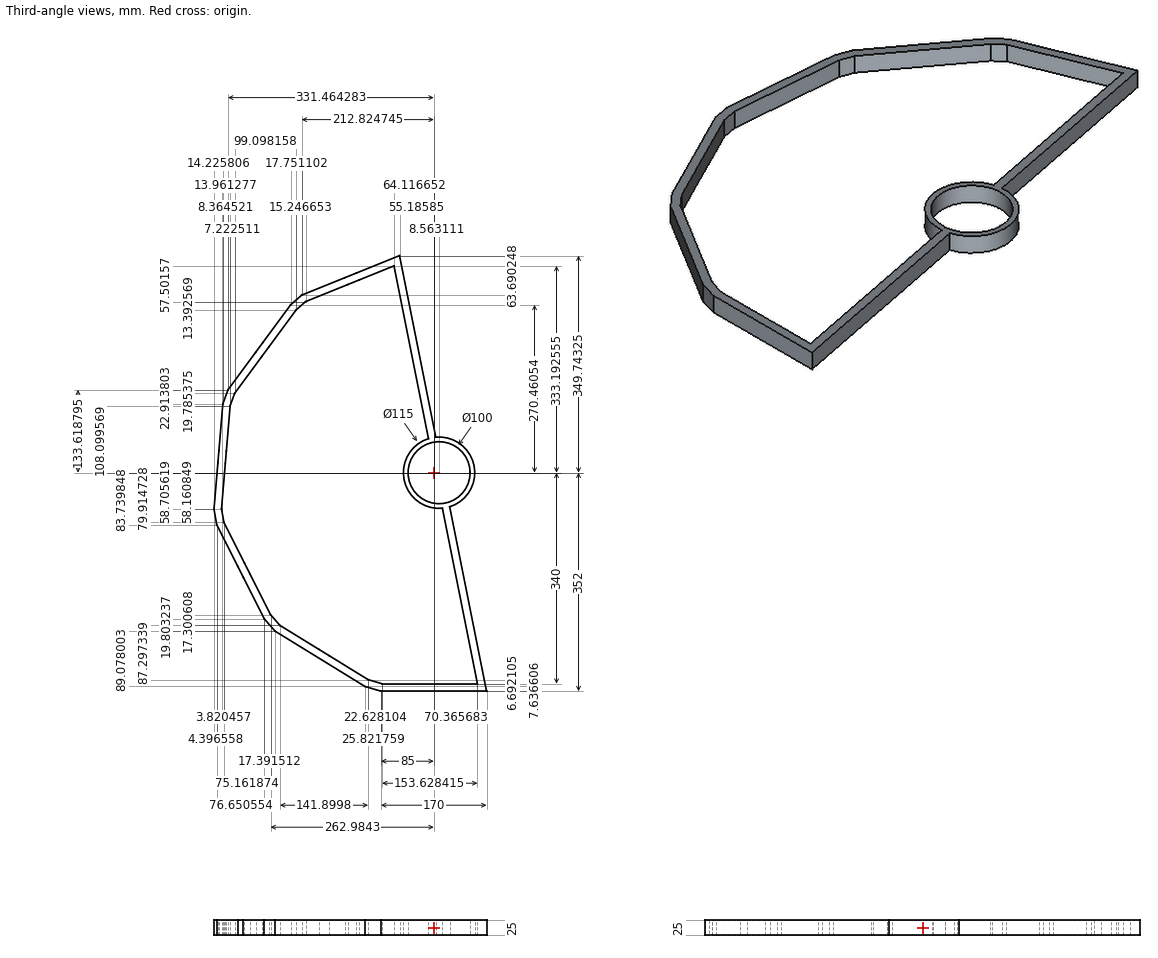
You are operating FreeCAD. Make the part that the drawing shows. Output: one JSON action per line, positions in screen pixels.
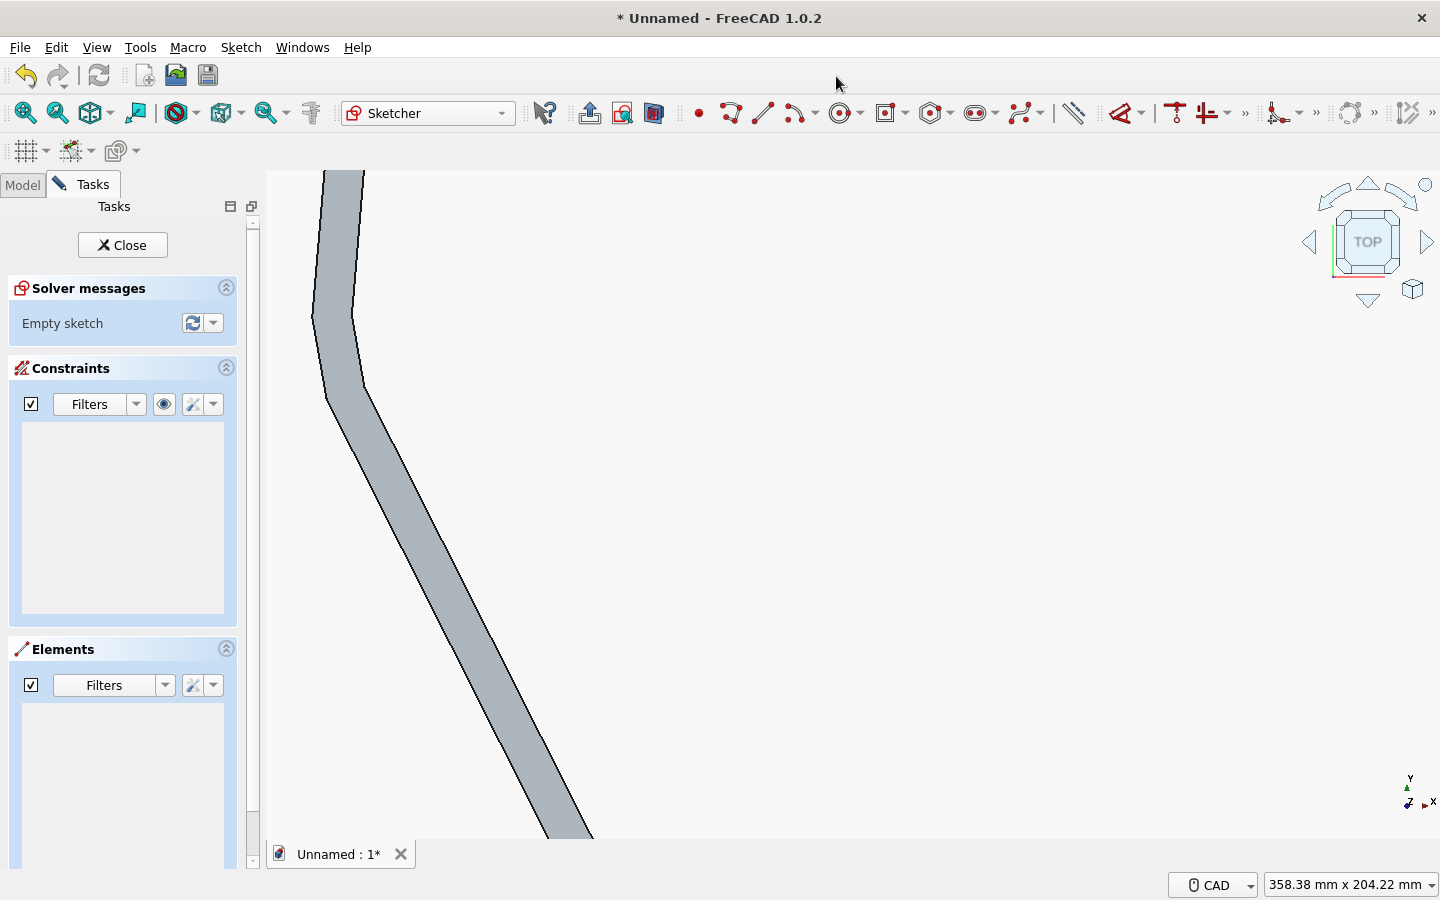
{"action": "scroll", "coordinate": [294, 811], "scroll_direction": "down", "scroll_amount": 2}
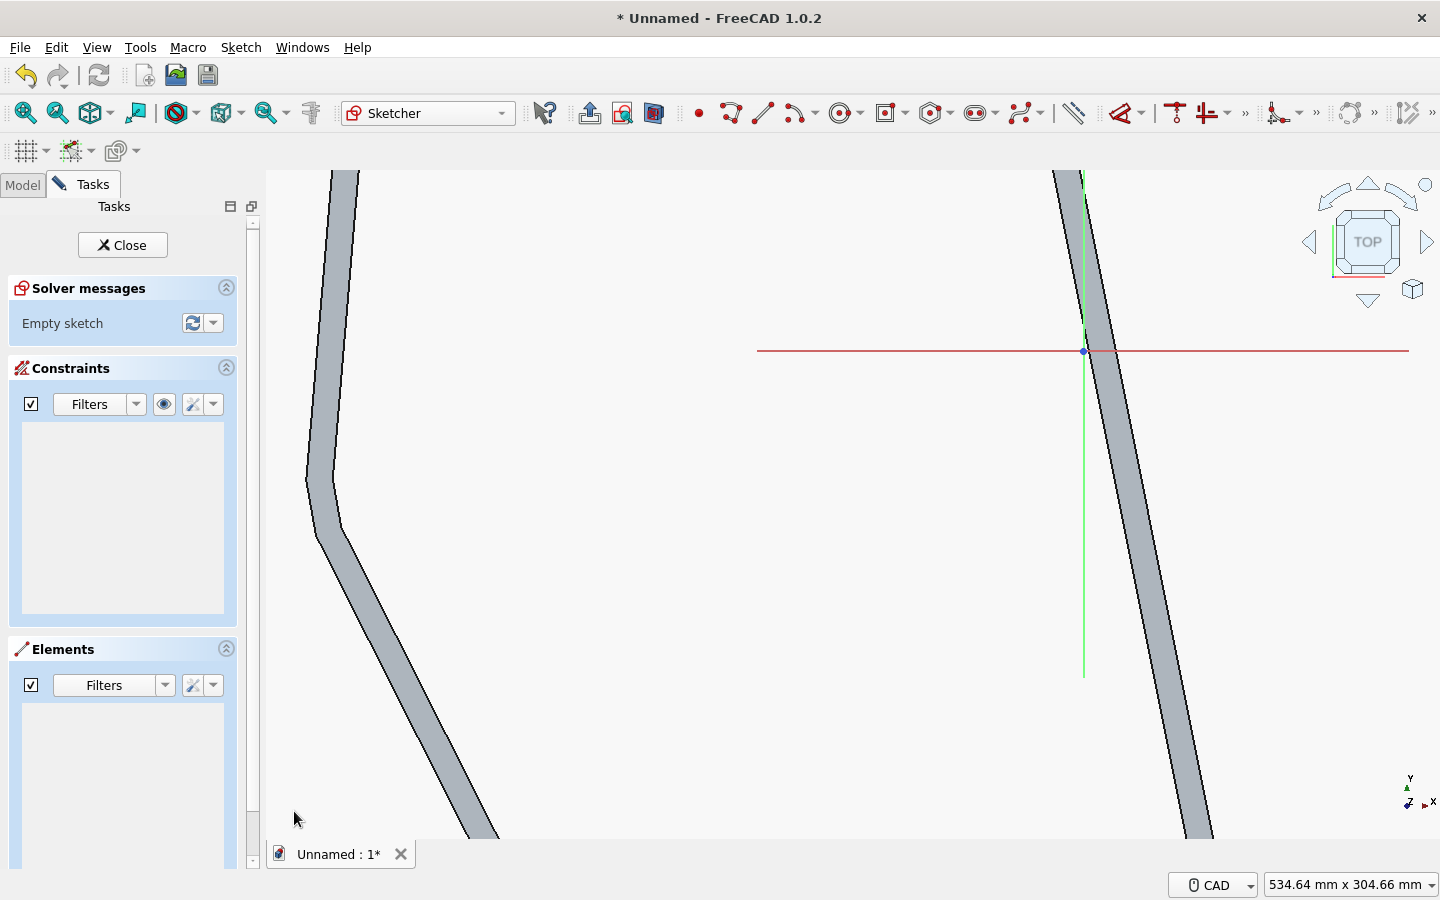
{"action": "scroll", "coordinate": [1275, 198], "scroll_direction": "up", "scroll_amount": 3}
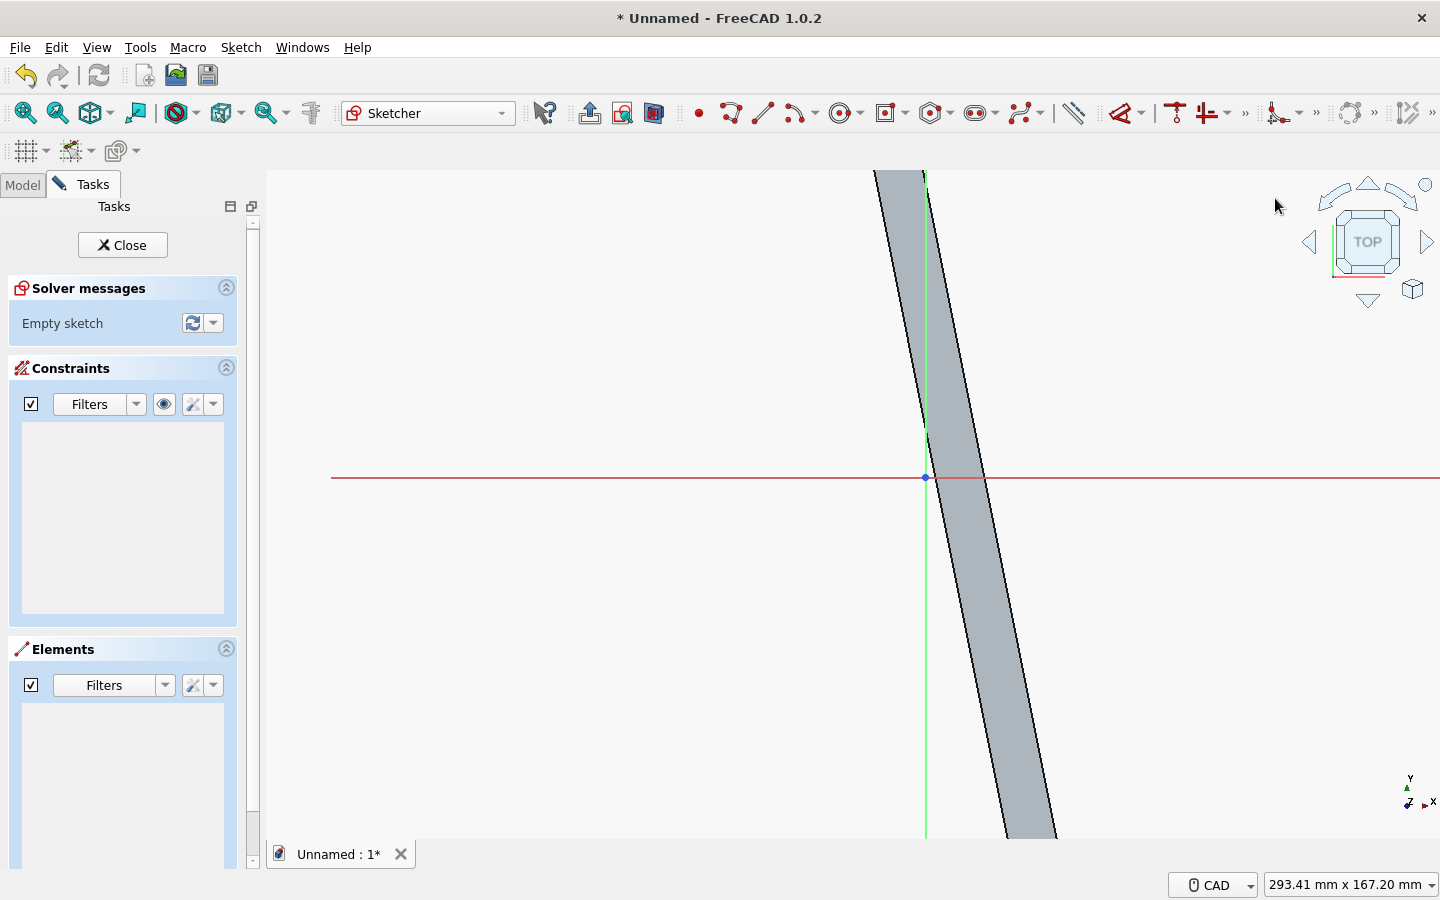
{"action": "left_click", "coordinate": [840, 114]}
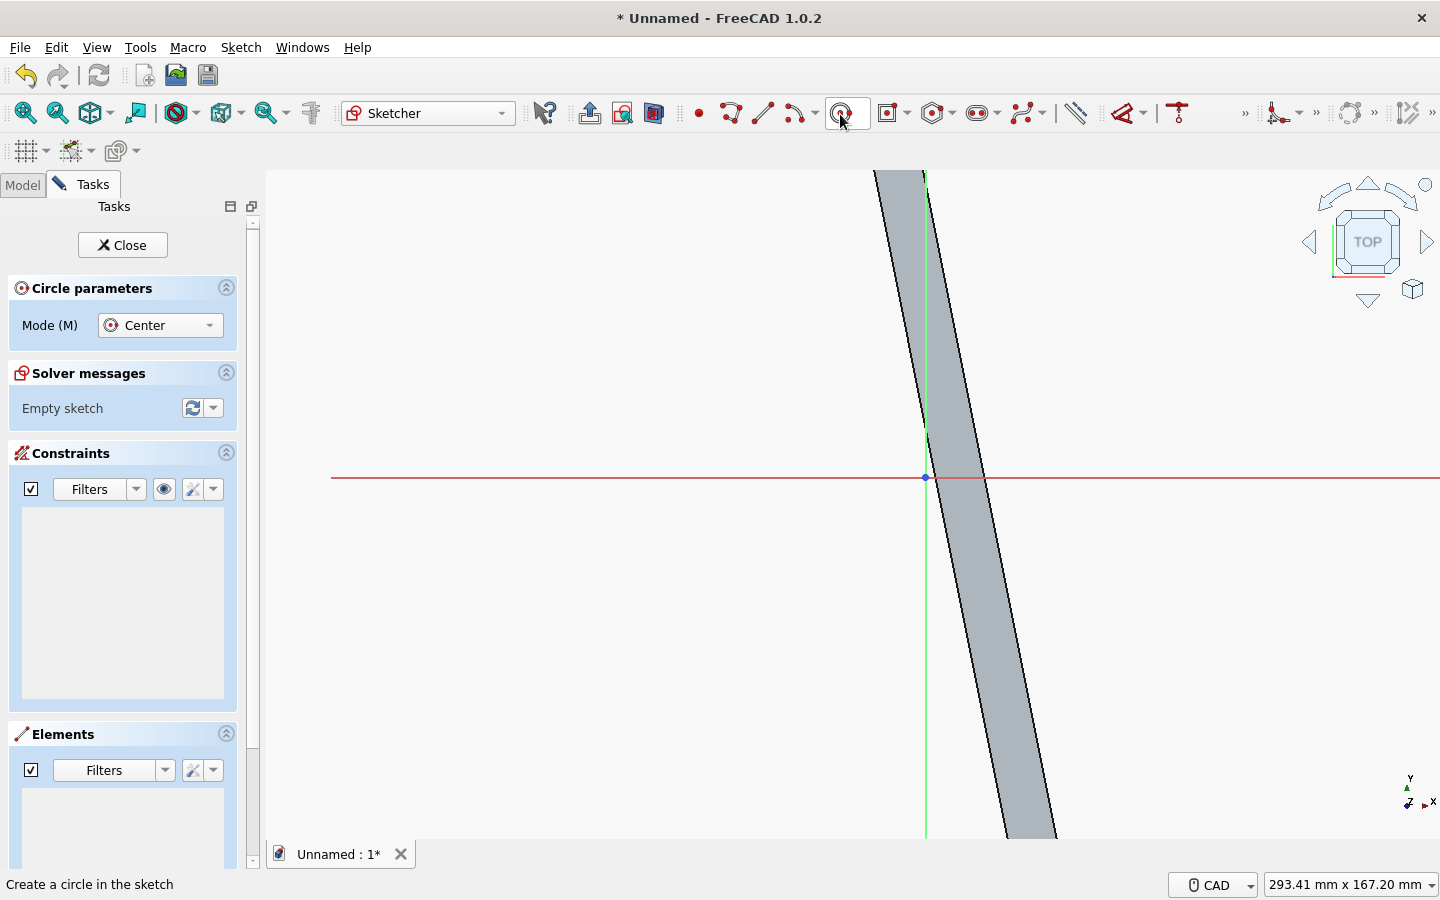
{"action": "left_click", "coordinate": [960, 478]}
{"action": "left_click", "coordinate": [1101, 336]}
{"action": "key", "text": "Escape"}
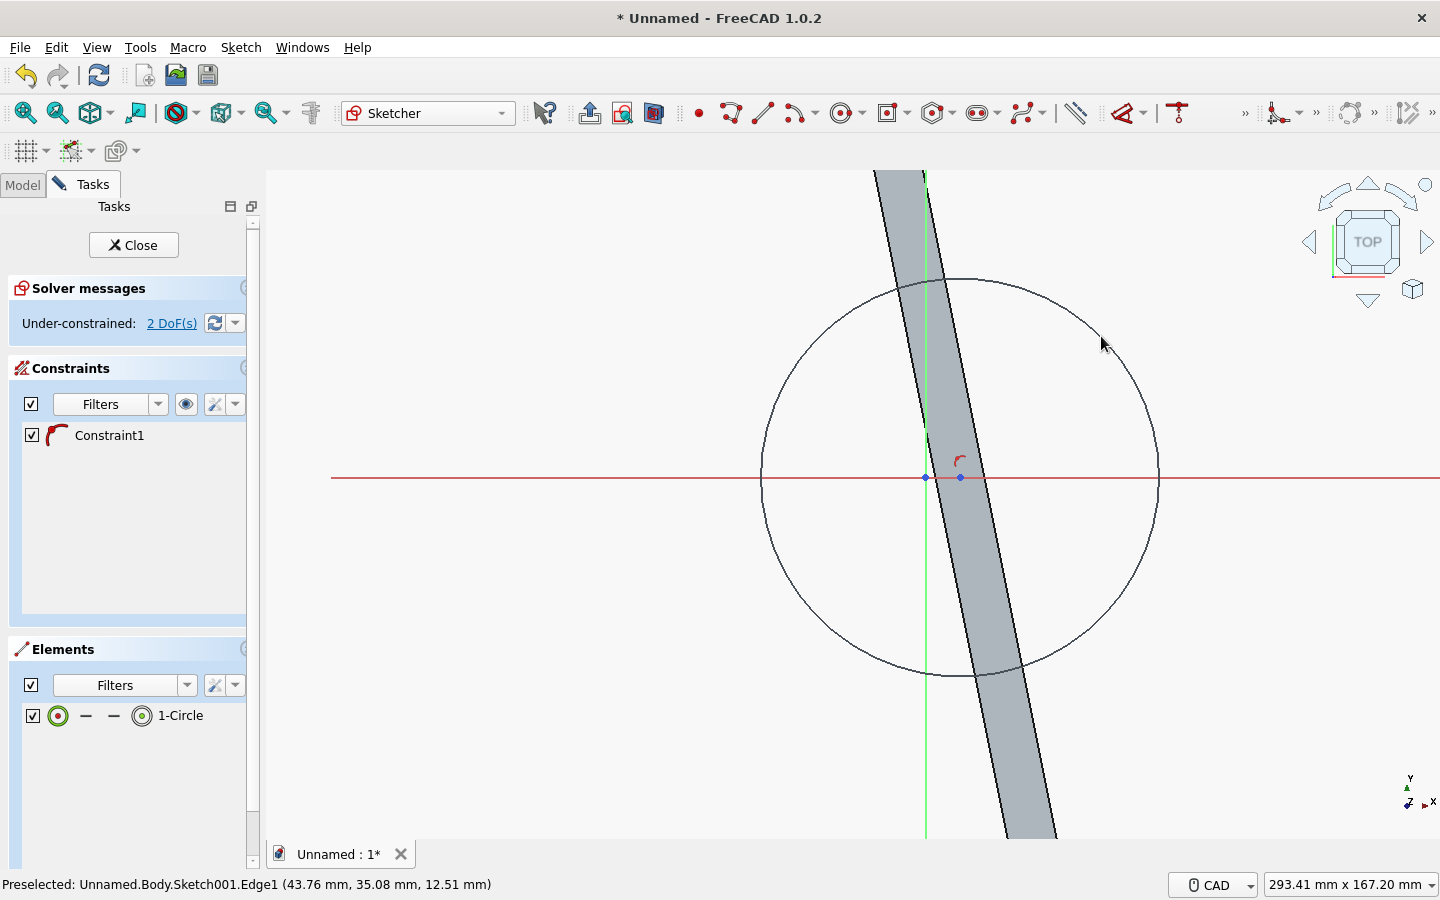
{"action": "left_click", "coordinate": [1122, 114]}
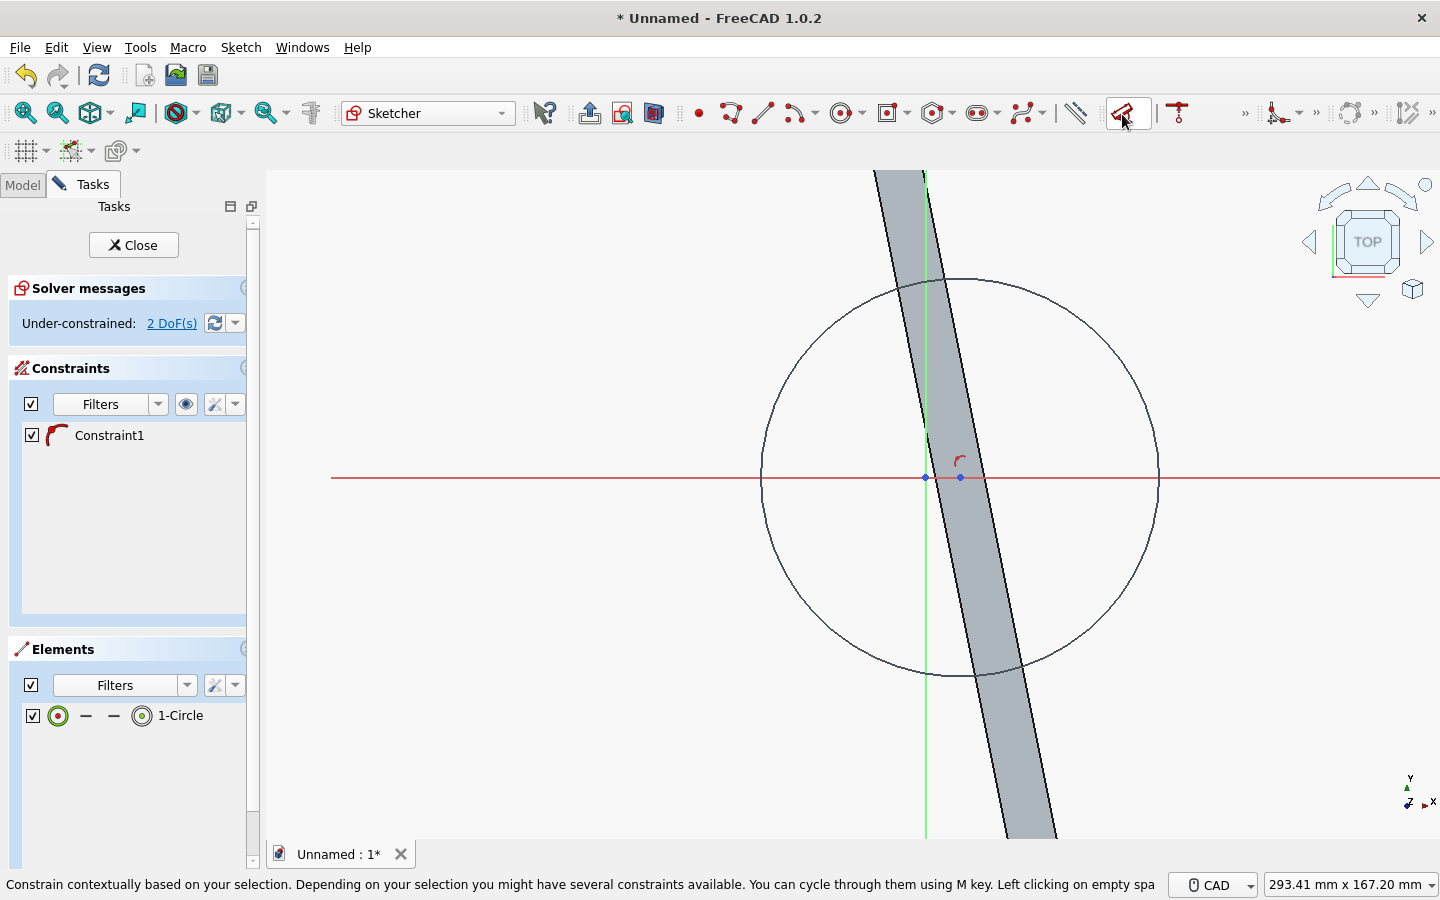
{"action": "left_click", "coordinate": [1100, 336]}
{"action": "left_click", "coordinate": [1122, 313]}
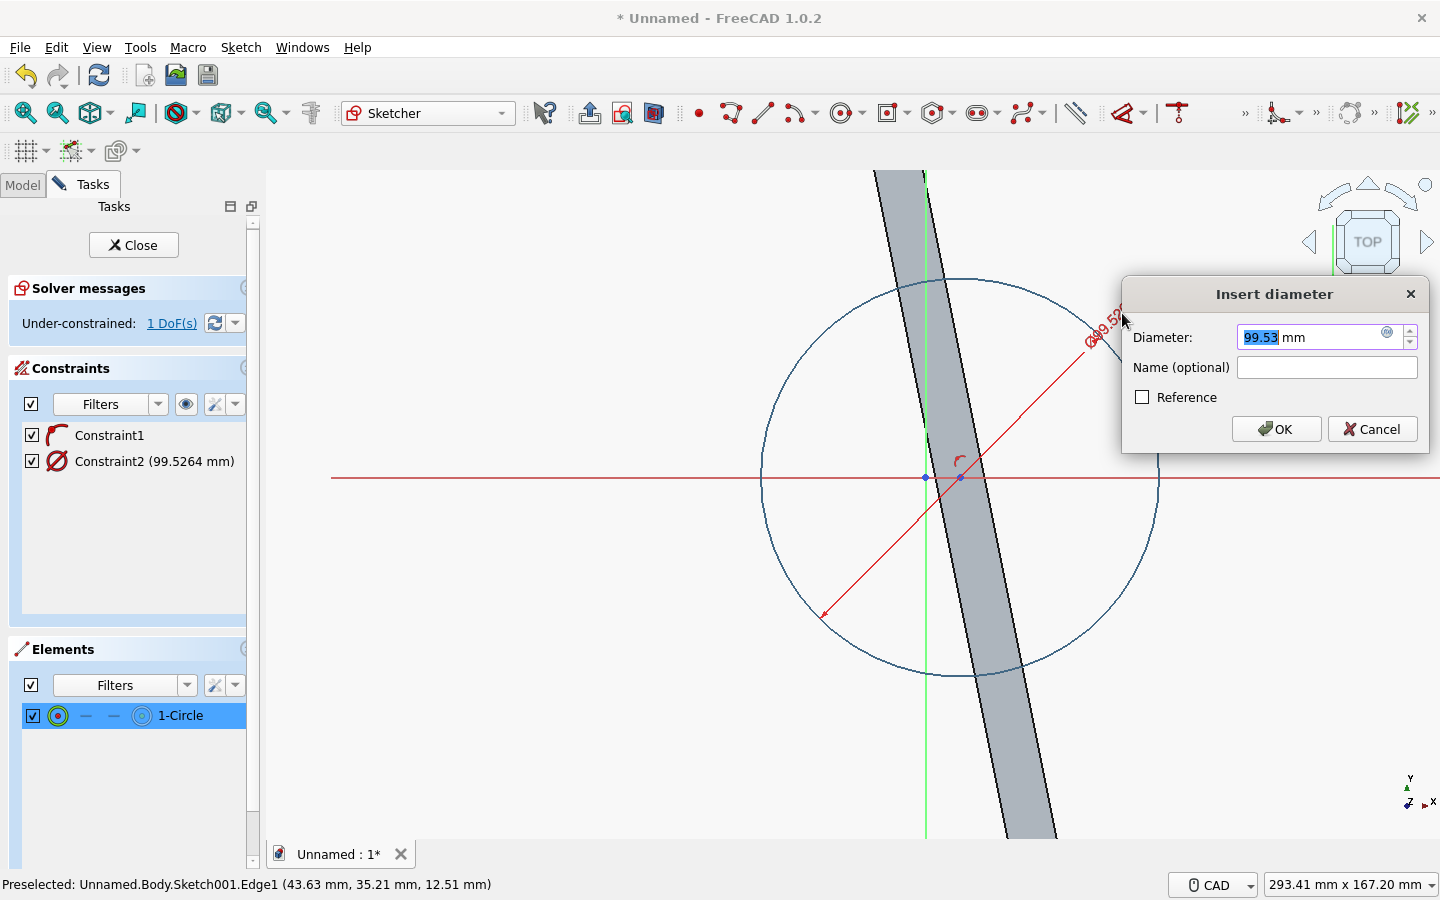
{"action": "type", "text": "100"}
{"action": "key", "text": "Return"}